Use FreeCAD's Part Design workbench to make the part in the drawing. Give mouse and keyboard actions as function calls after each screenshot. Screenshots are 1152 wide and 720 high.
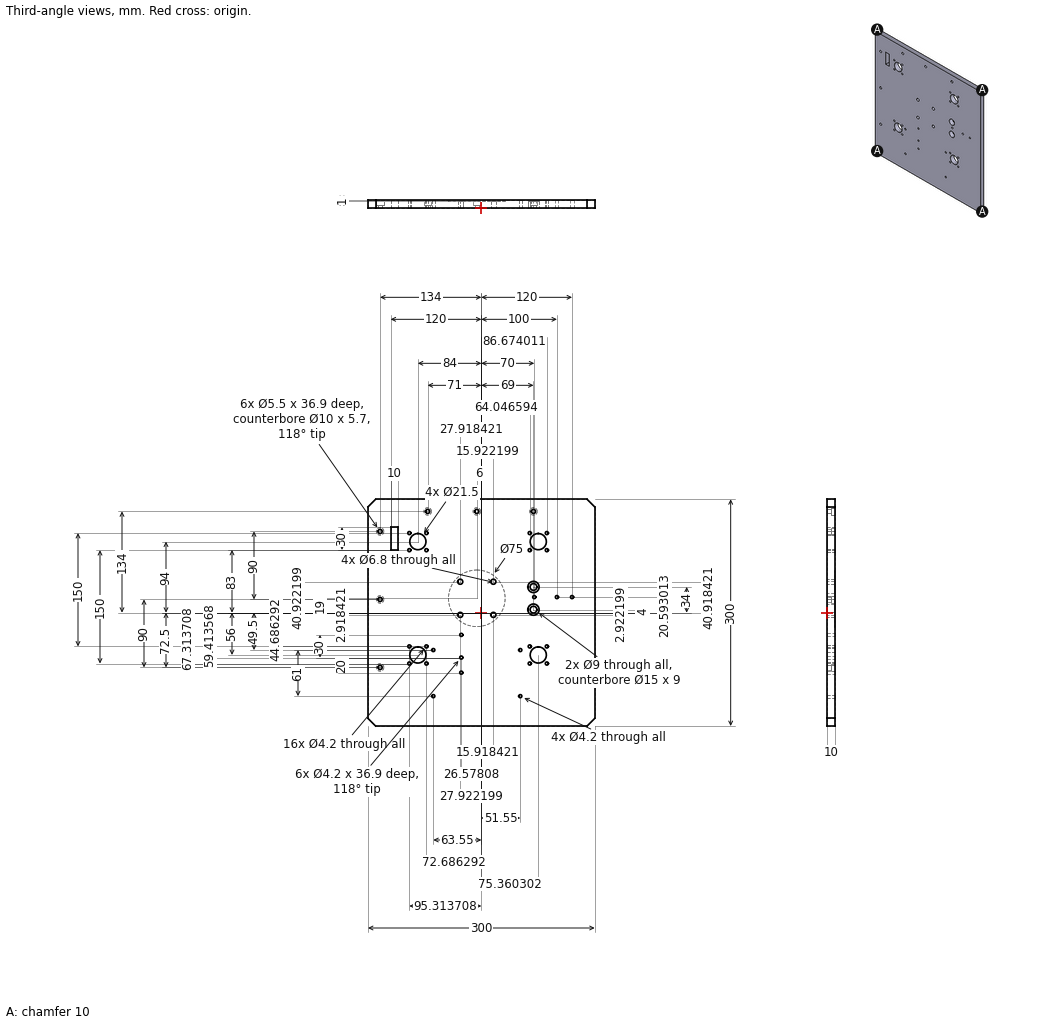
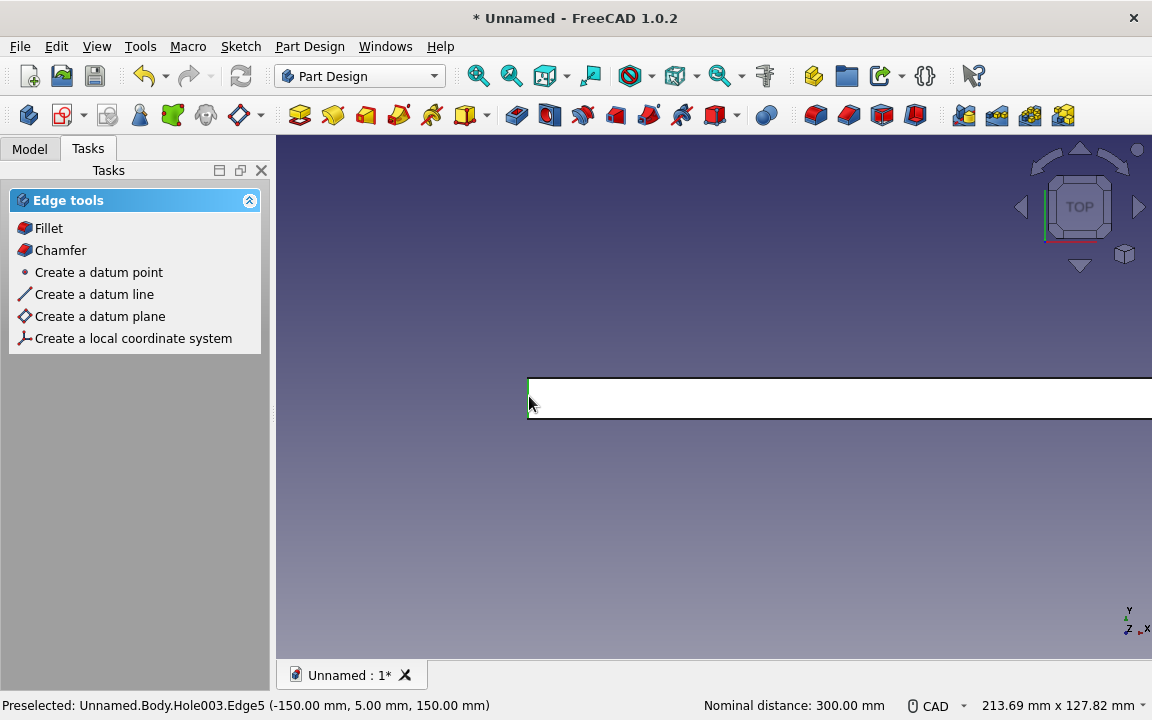
click(479, 76)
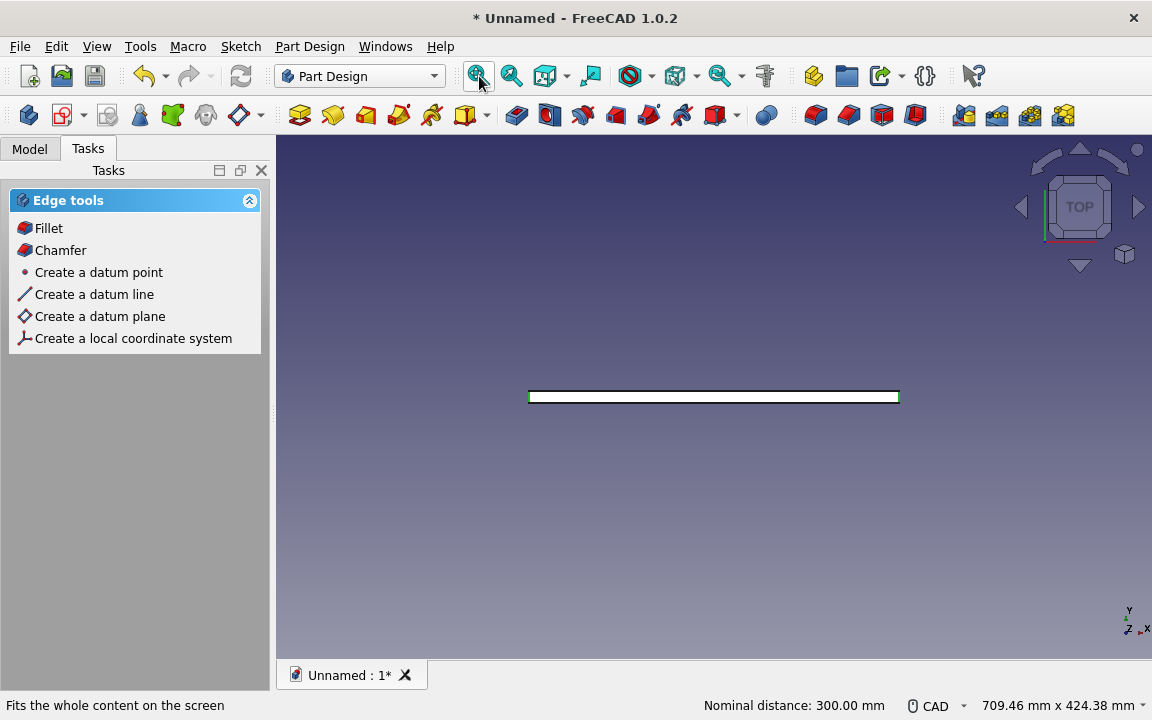
key(1)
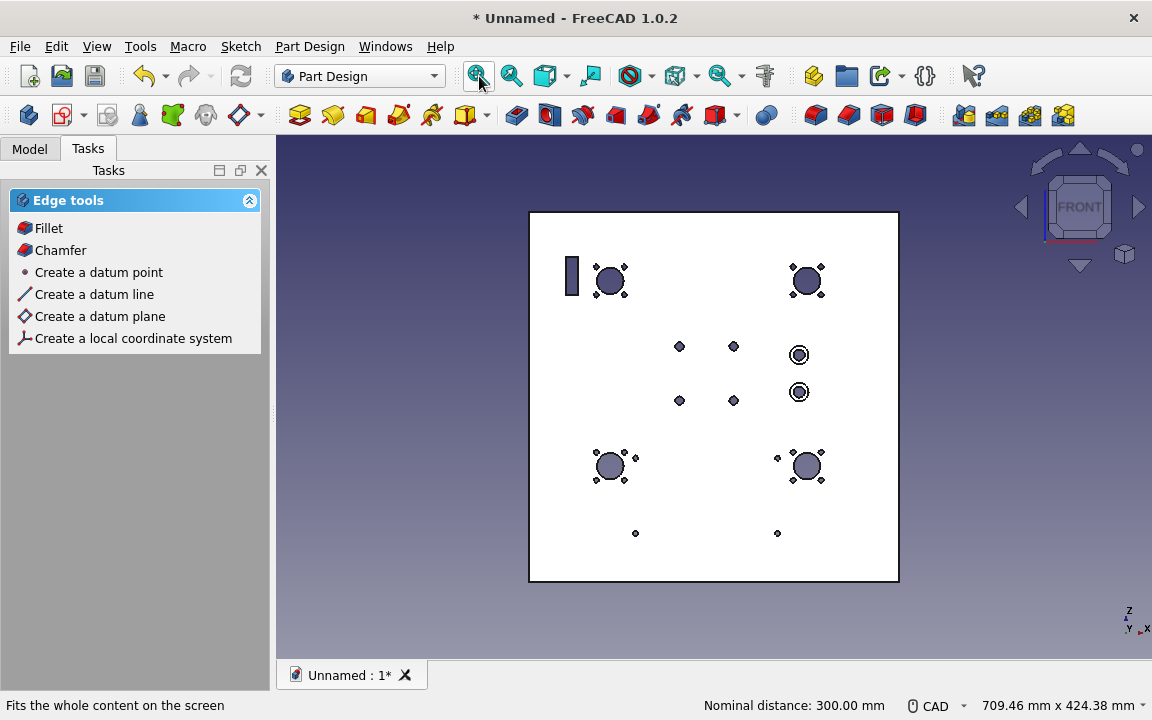
scroll(529, 581, up, 6)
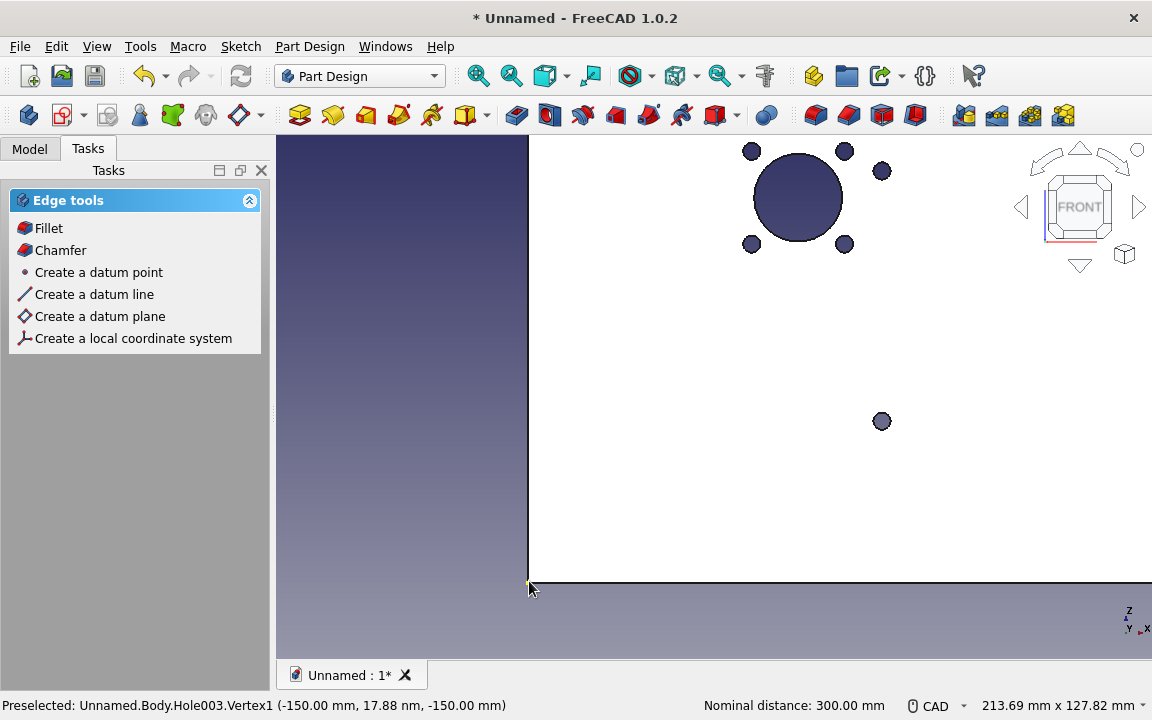
click(479, 76)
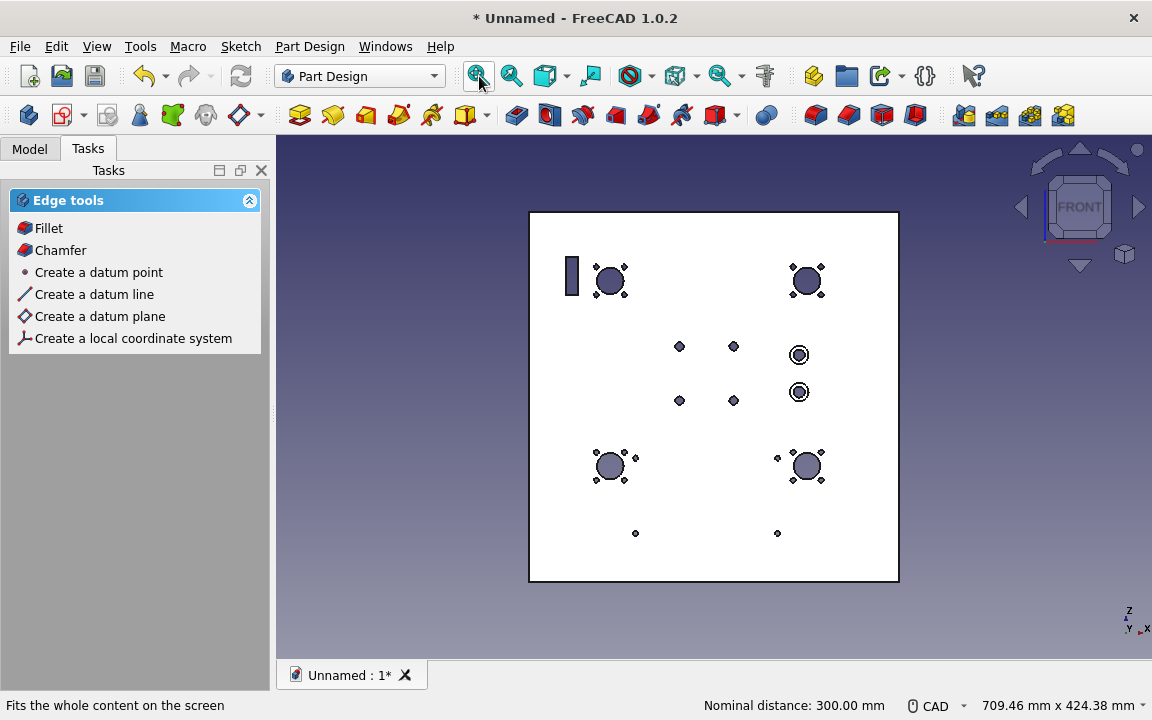
key(3)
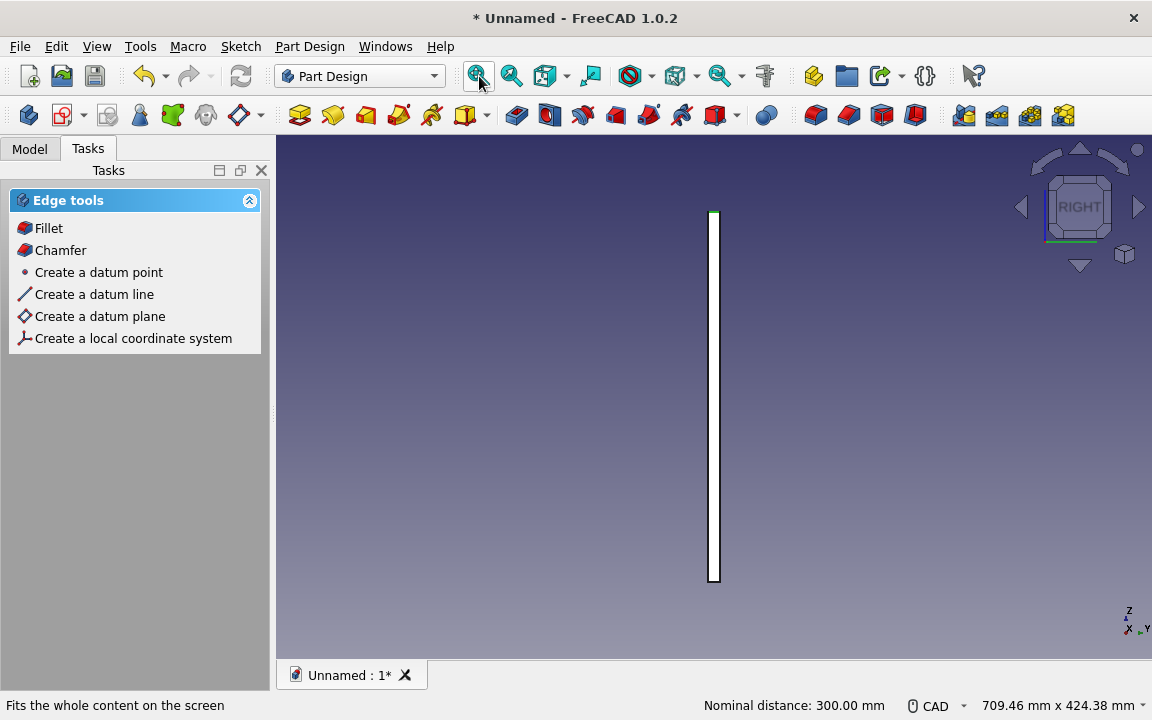
click(714, 581, ctrl)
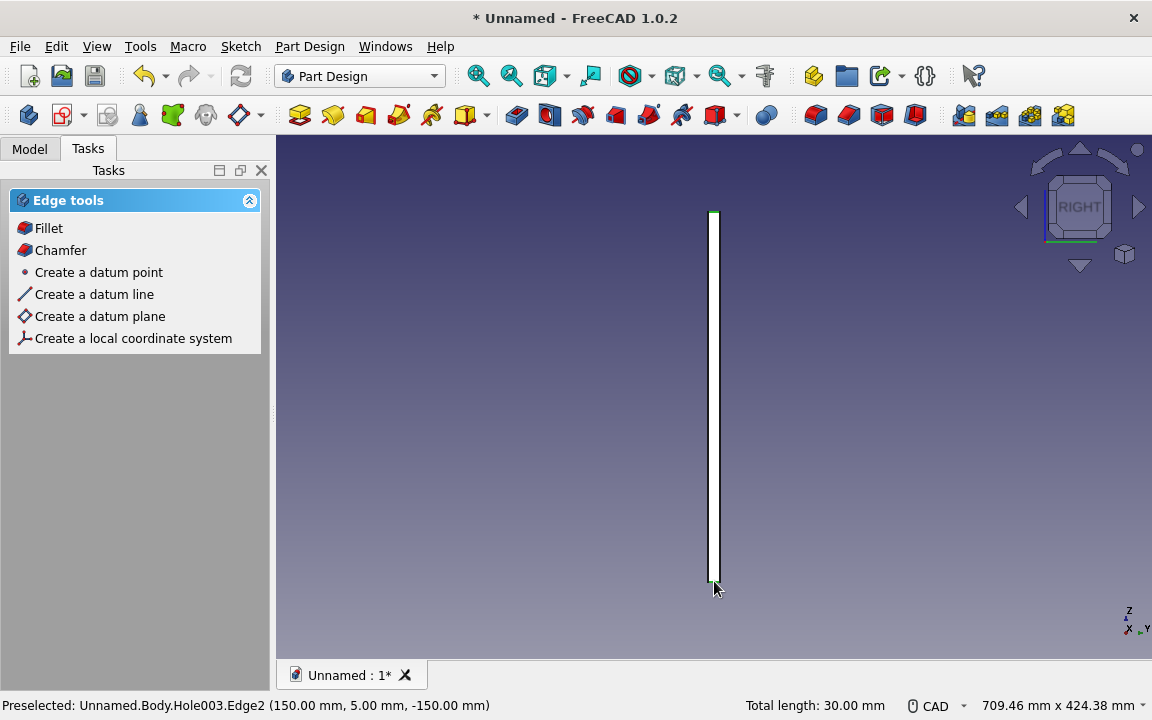
scroll(714, 581, up, 6)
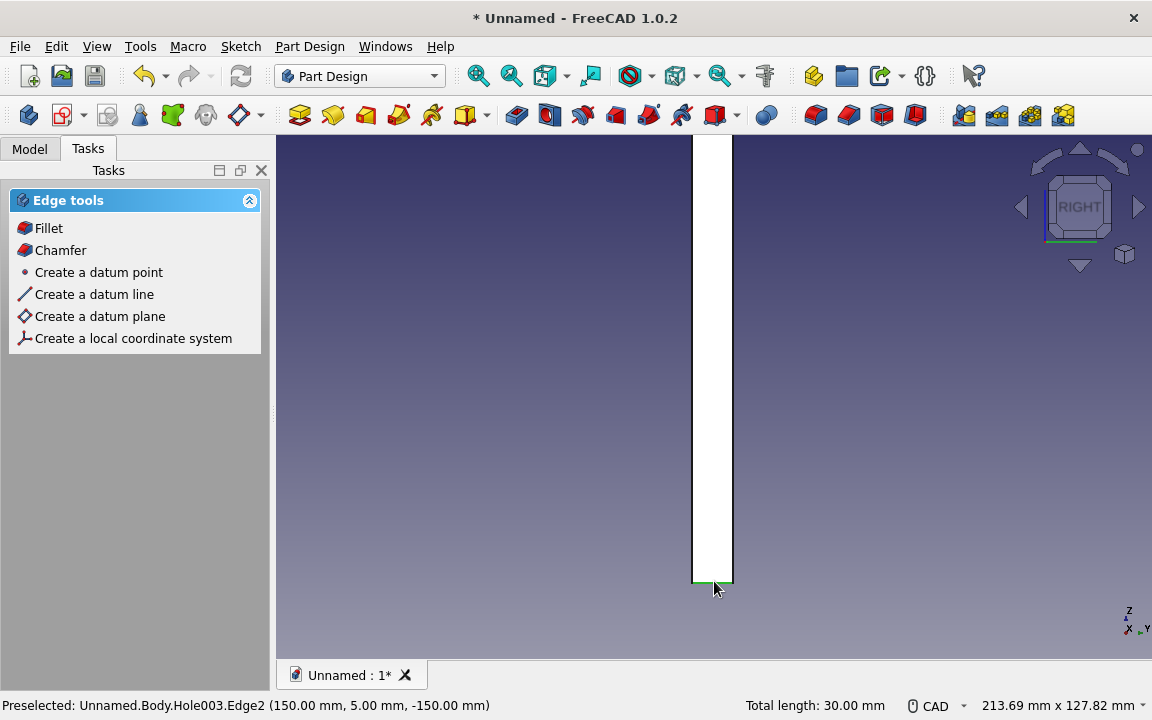
click(479, 76)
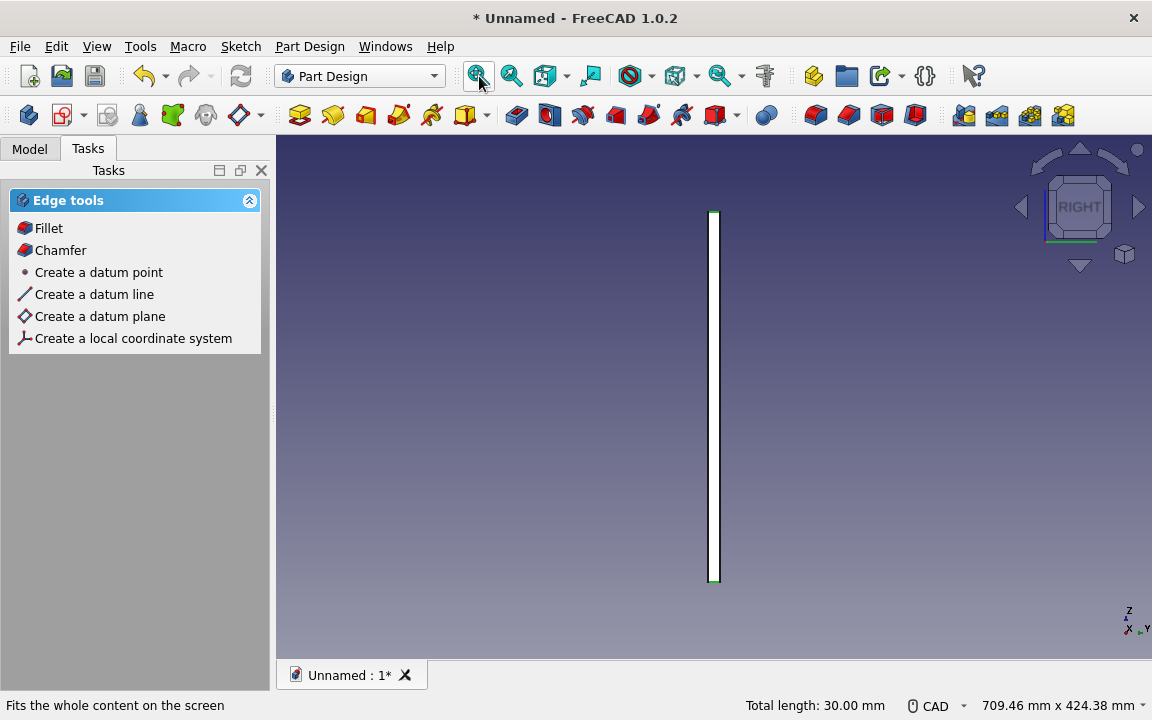
key(5)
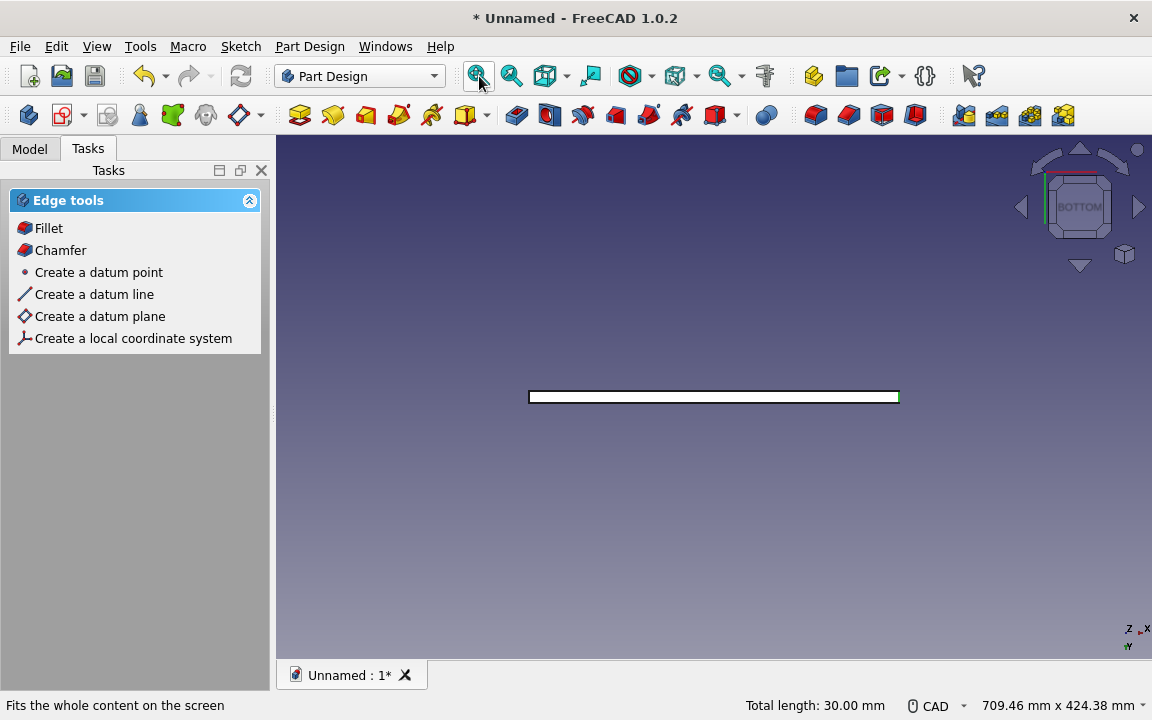
click(479, 76)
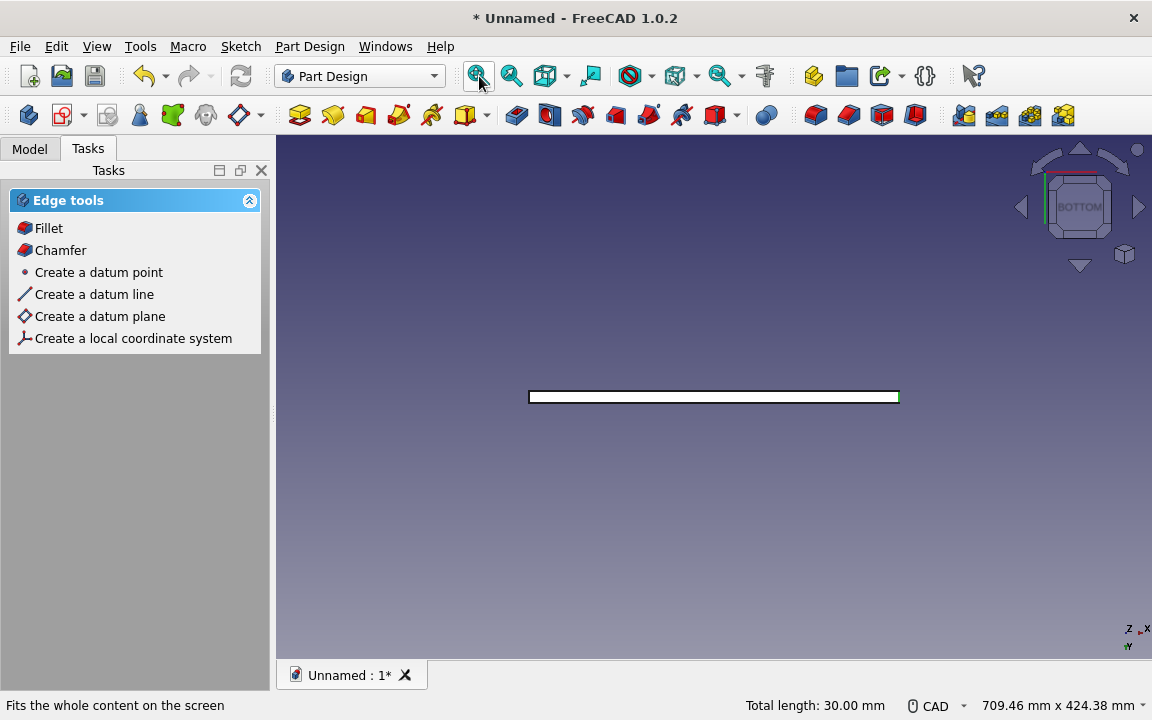
click(529, 396, ctrl)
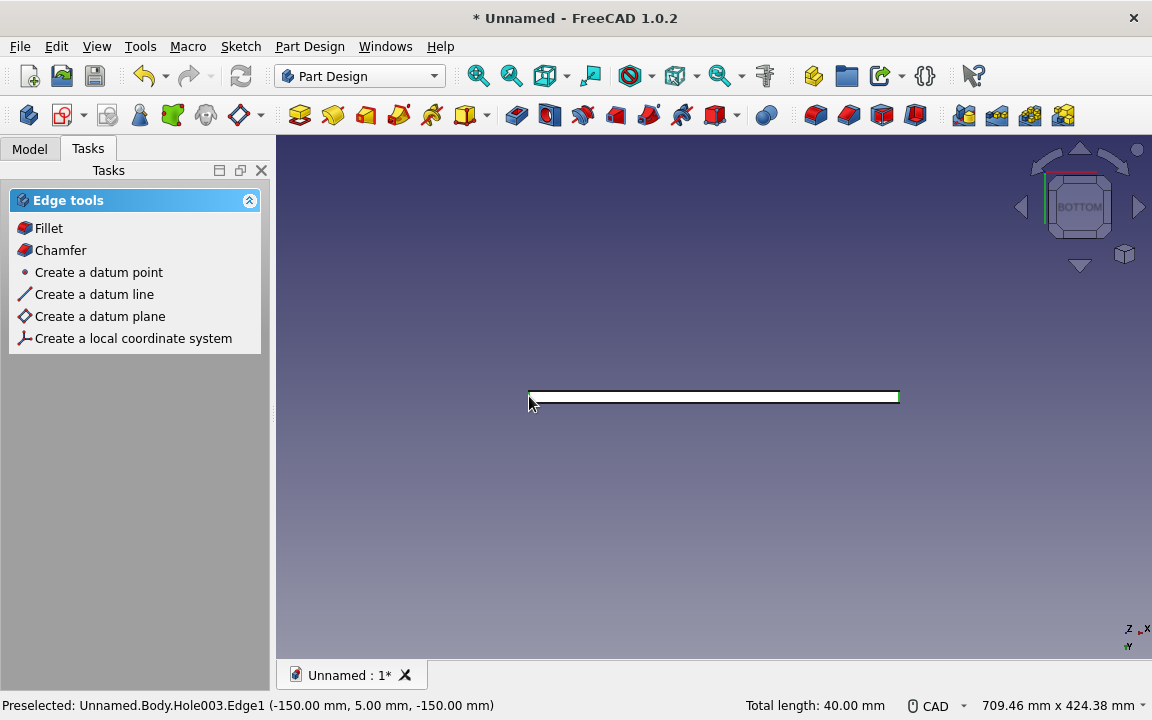
click(849, 116)